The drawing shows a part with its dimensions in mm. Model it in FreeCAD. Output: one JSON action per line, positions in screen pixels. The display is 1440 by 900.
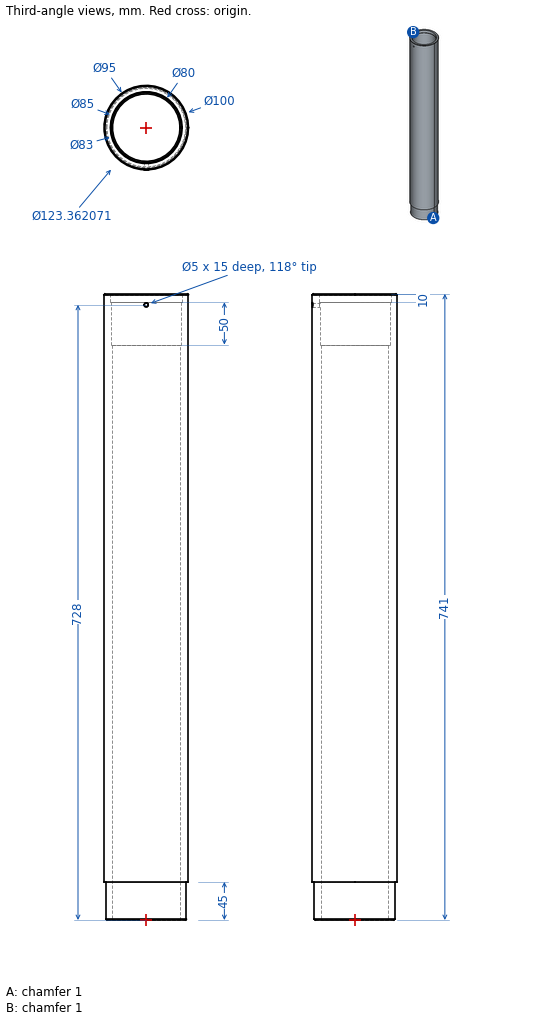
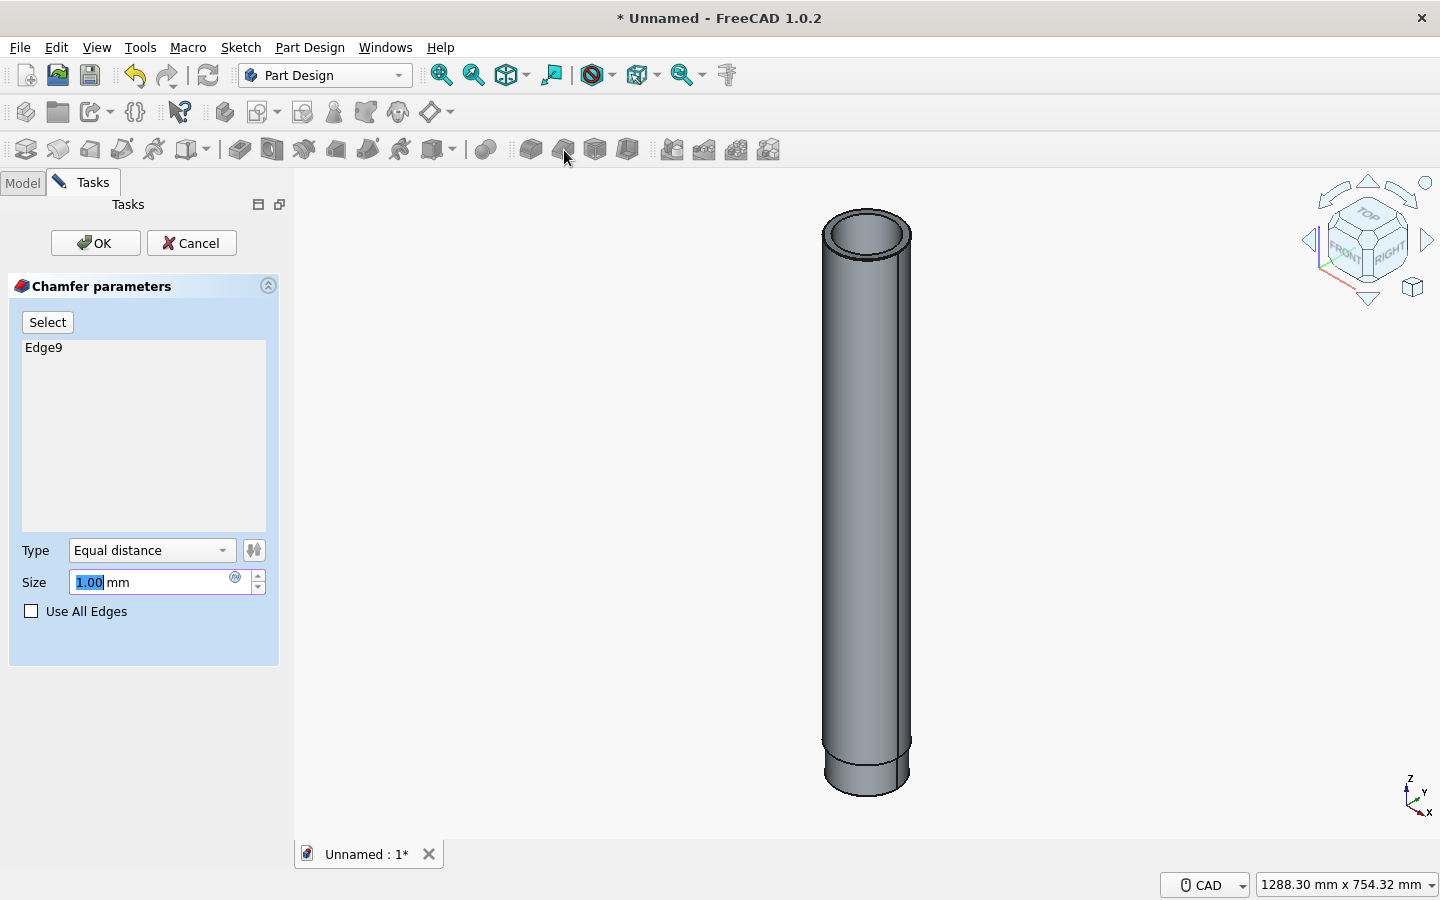
{"action": "type", "text": "1"}
{"action": "key", "text": "Tab"}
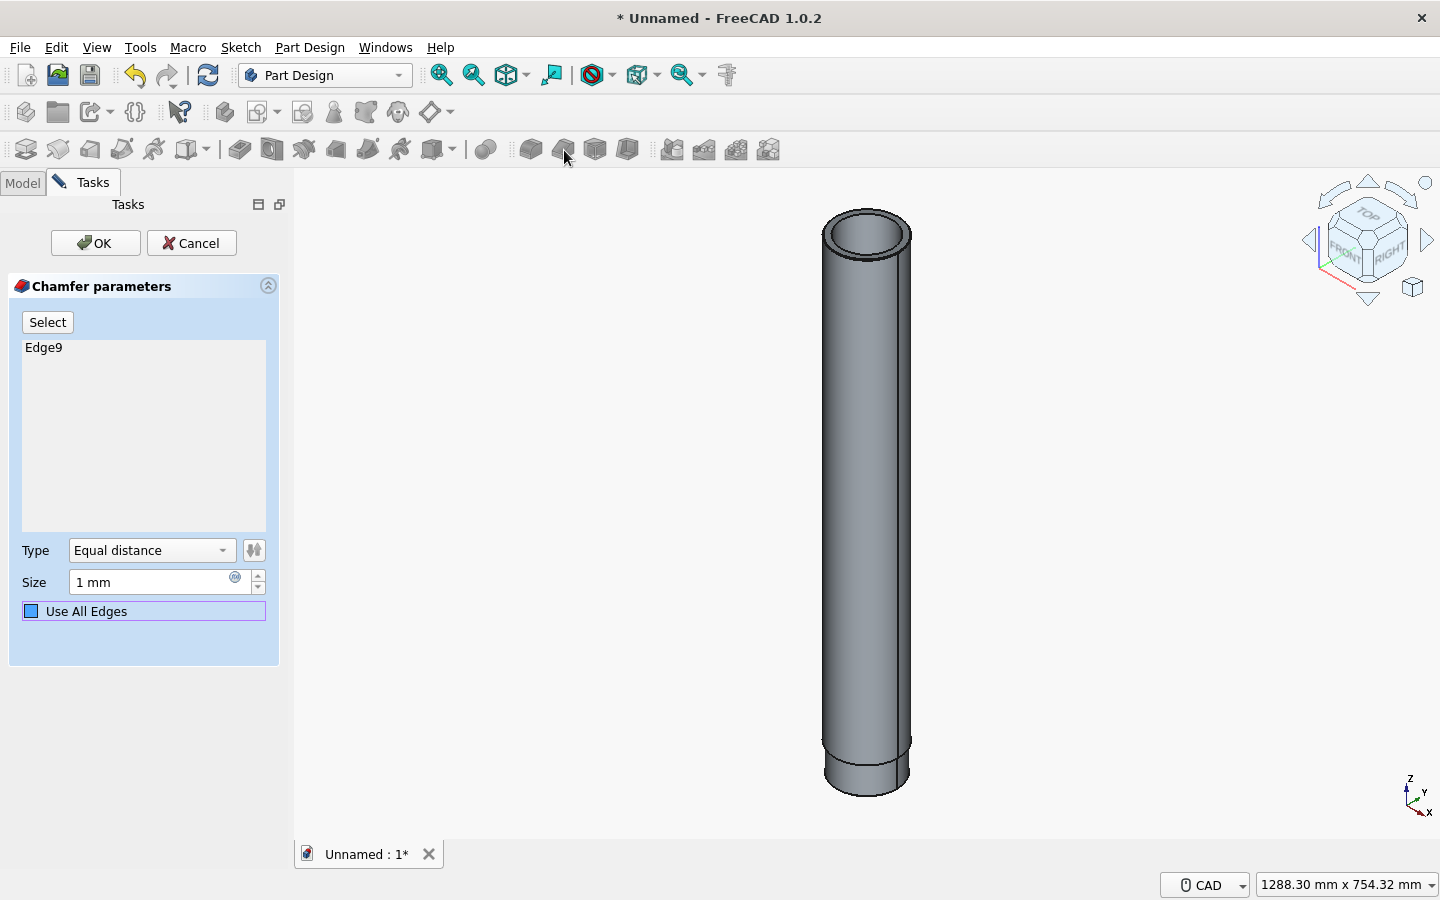
{"action": "left_click", "coordinate": [96, 243]}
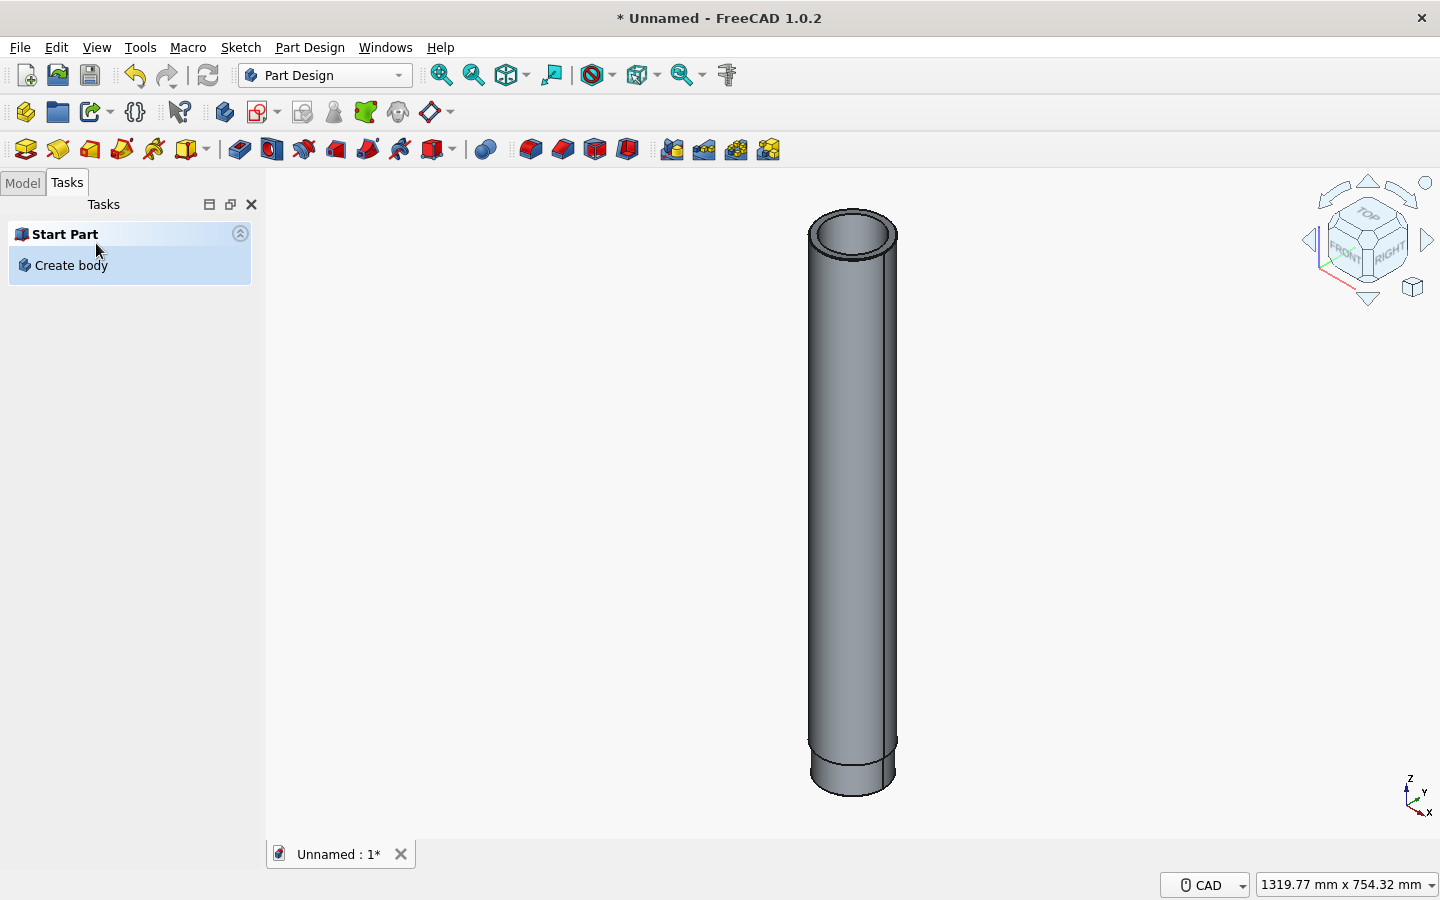
{"action": "scroll", "coordinate": [835, 254], "scroll_direction": "up", "scroll_amount": 6}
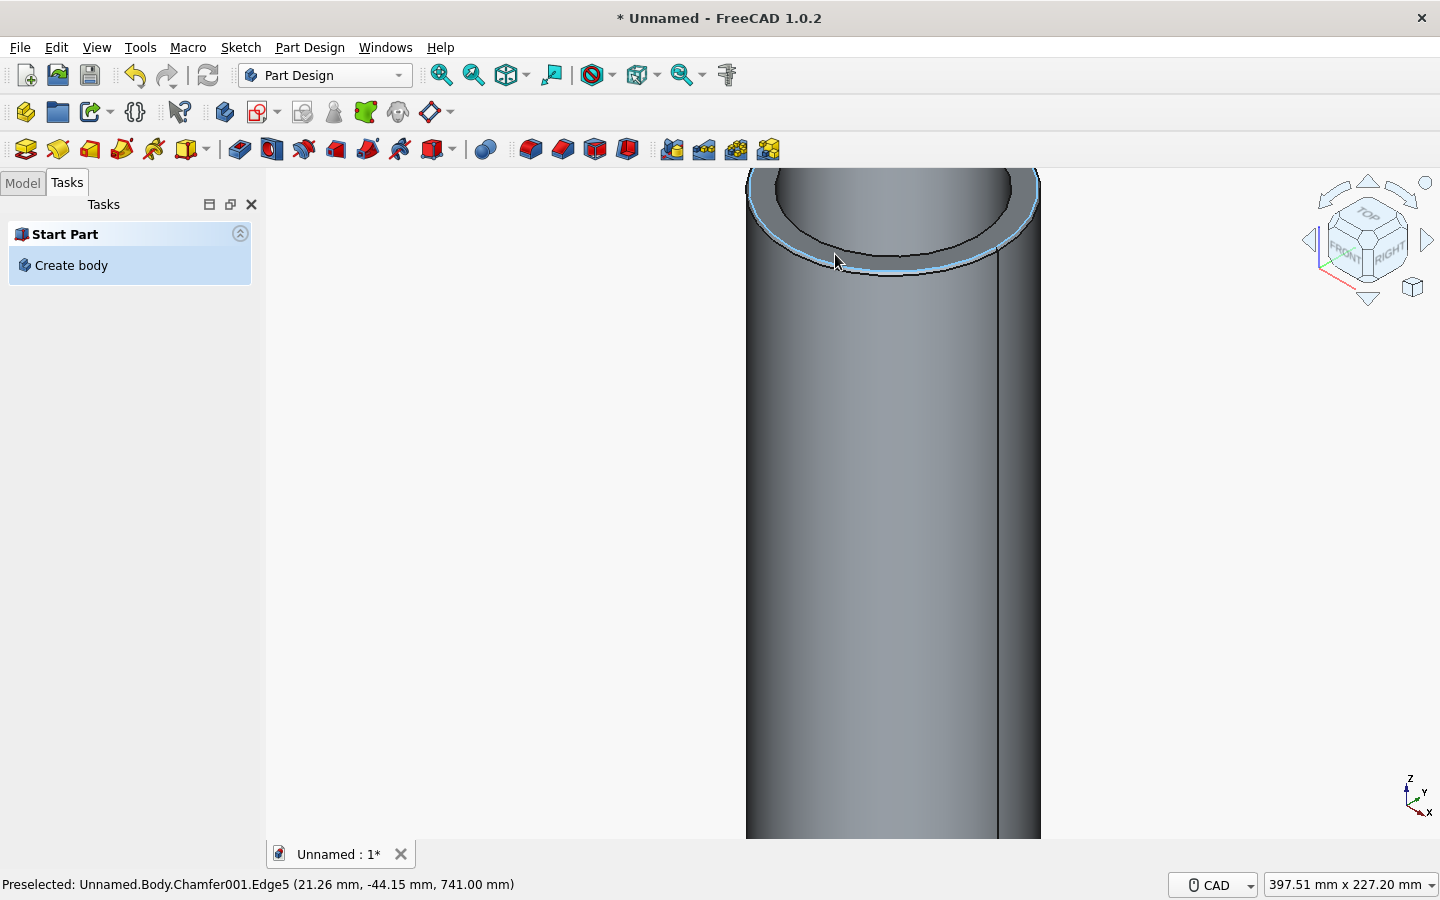
{"action": "left_click", "coordinate": [1010, 221]}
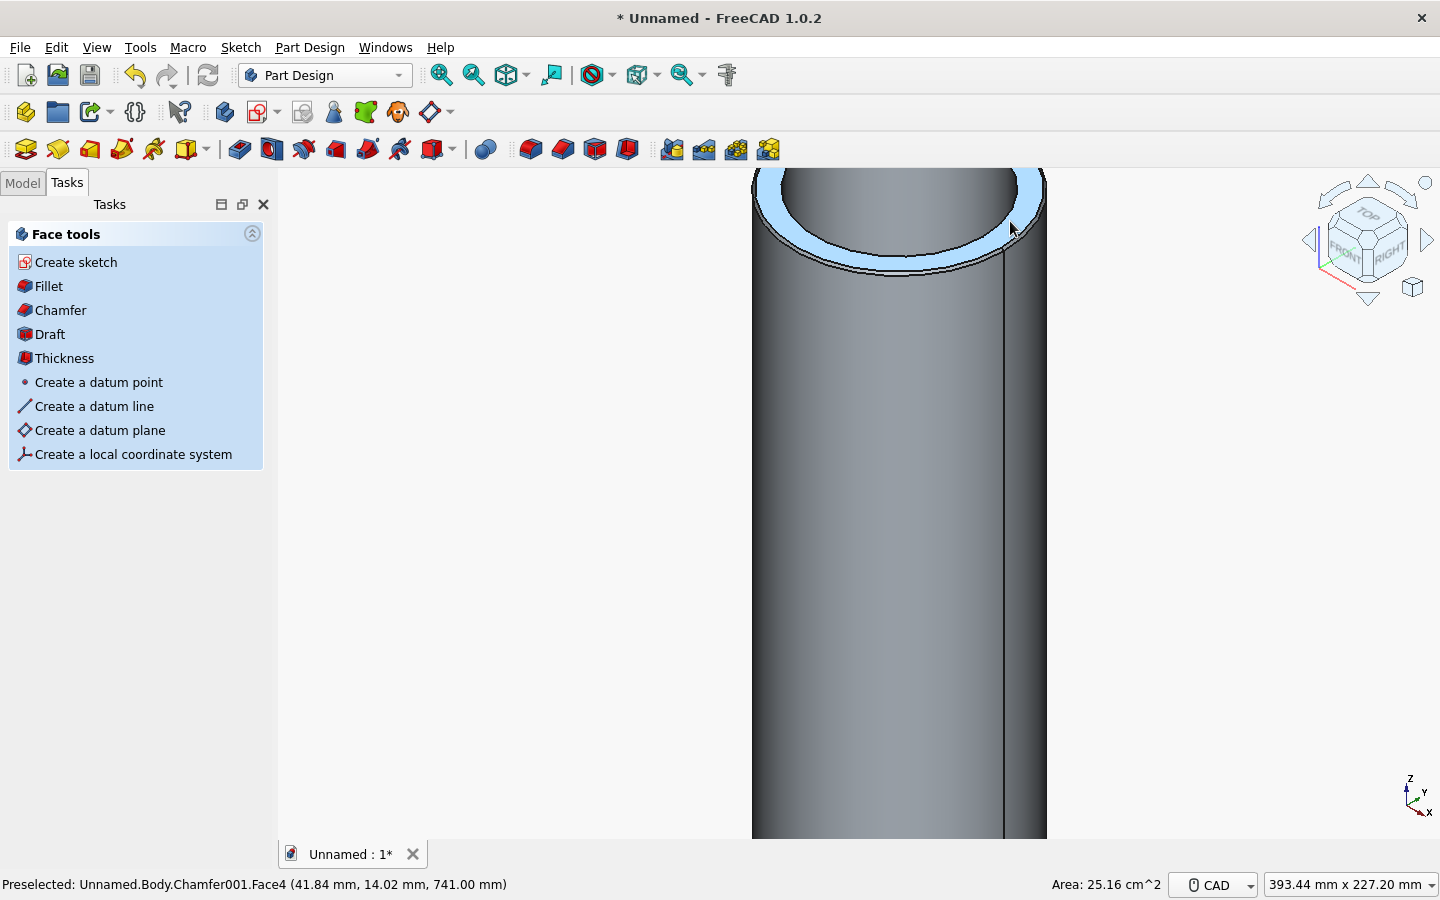
{"action": "left_click", "coordinate": [258, 112]}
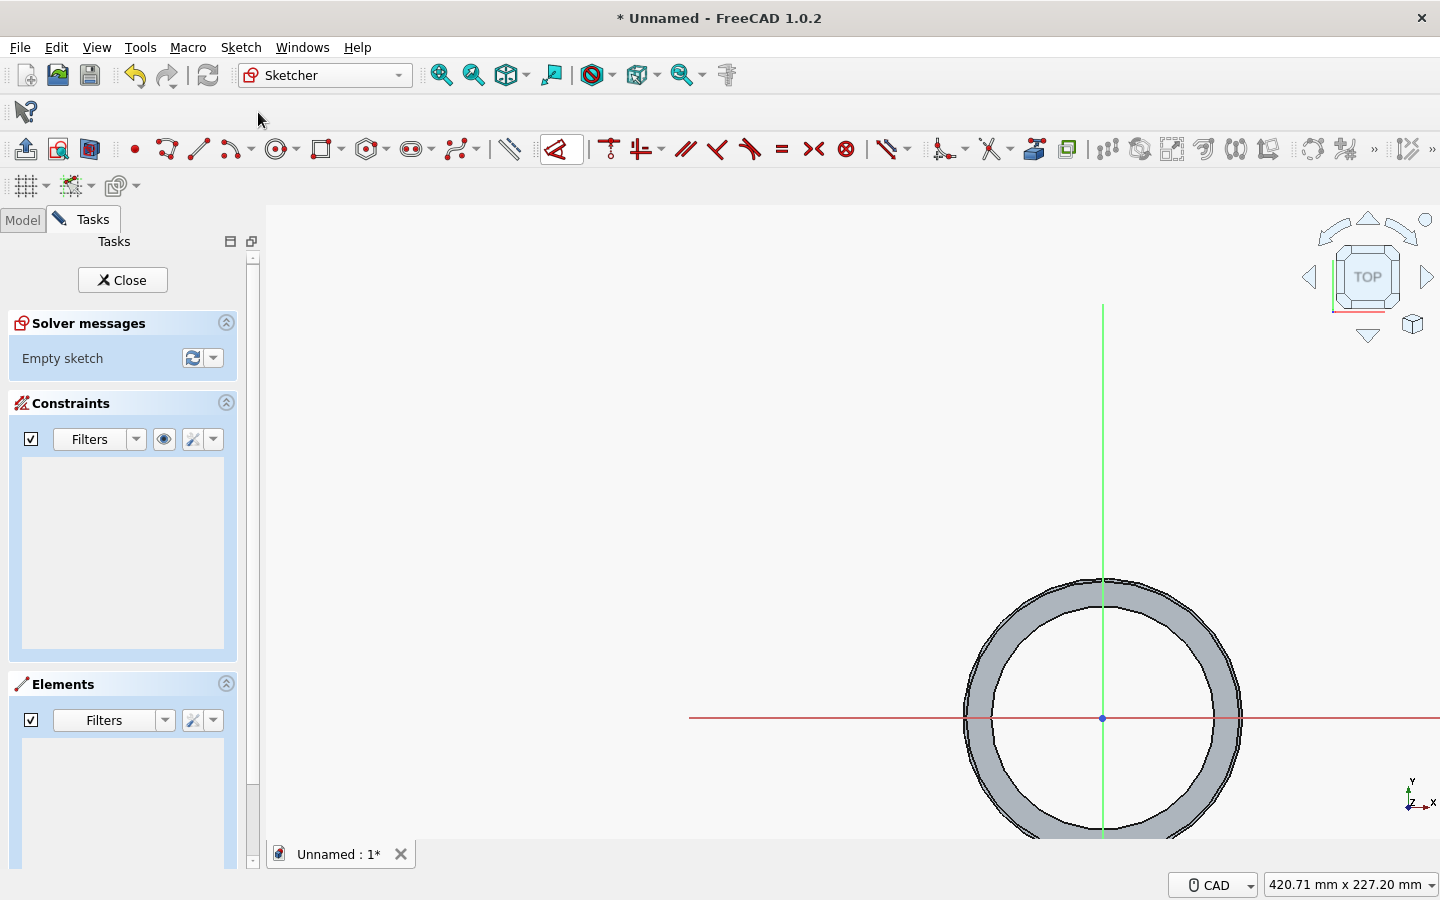
{"action": "scroll", "coordinate": [784, 522], "scroll_direction": "down", "scroll_amount": 5}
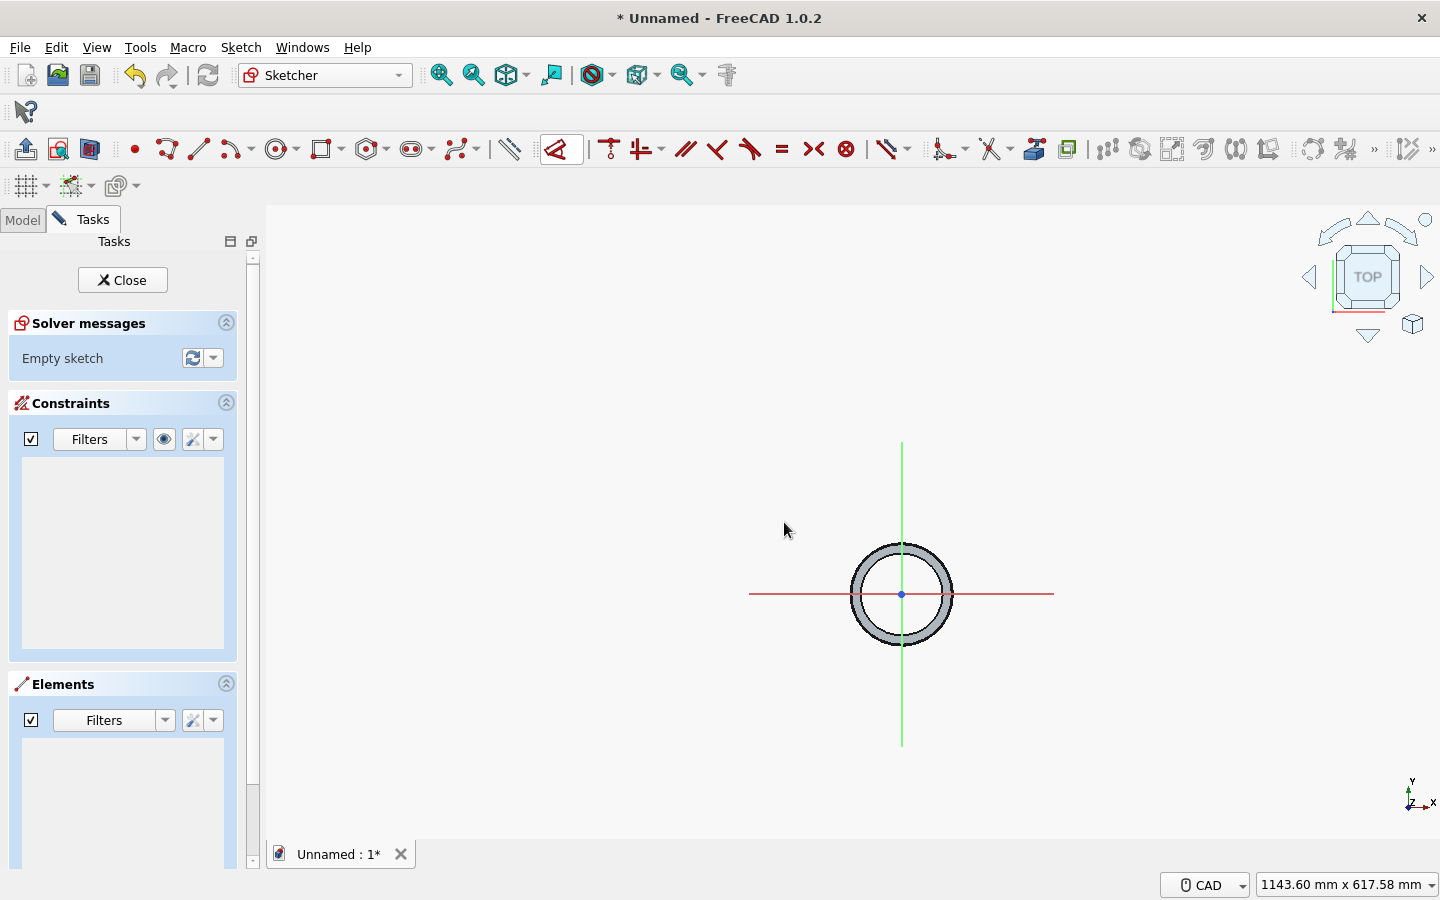
{"action": "scroll", "coordinate": [931, 613], "scroll_direction": "up", "scroll_amount": 8}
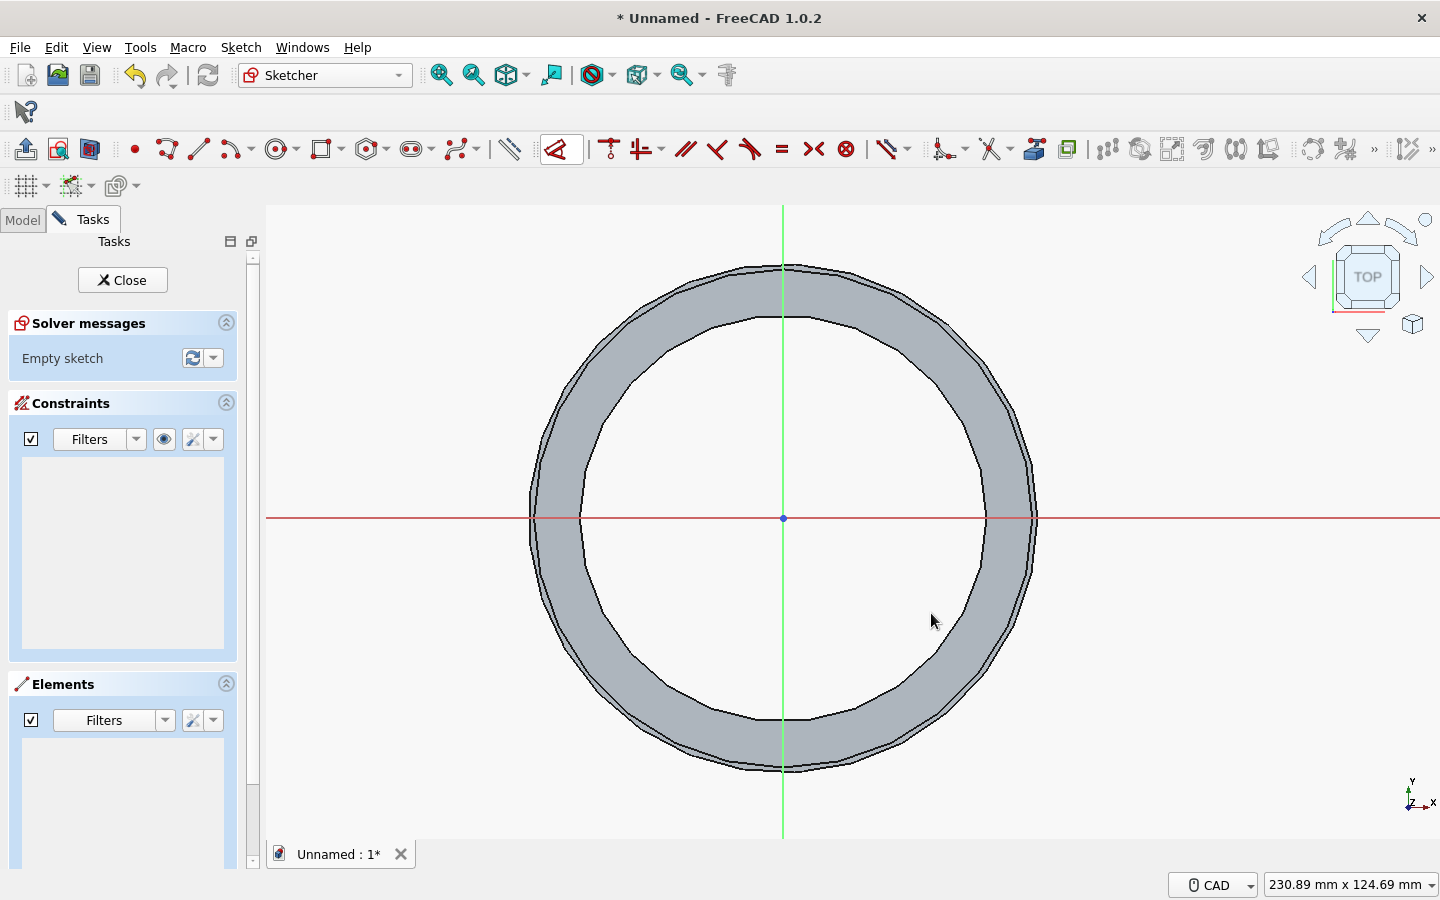
{"action": "left_click", "coordinate": [276, 150]}